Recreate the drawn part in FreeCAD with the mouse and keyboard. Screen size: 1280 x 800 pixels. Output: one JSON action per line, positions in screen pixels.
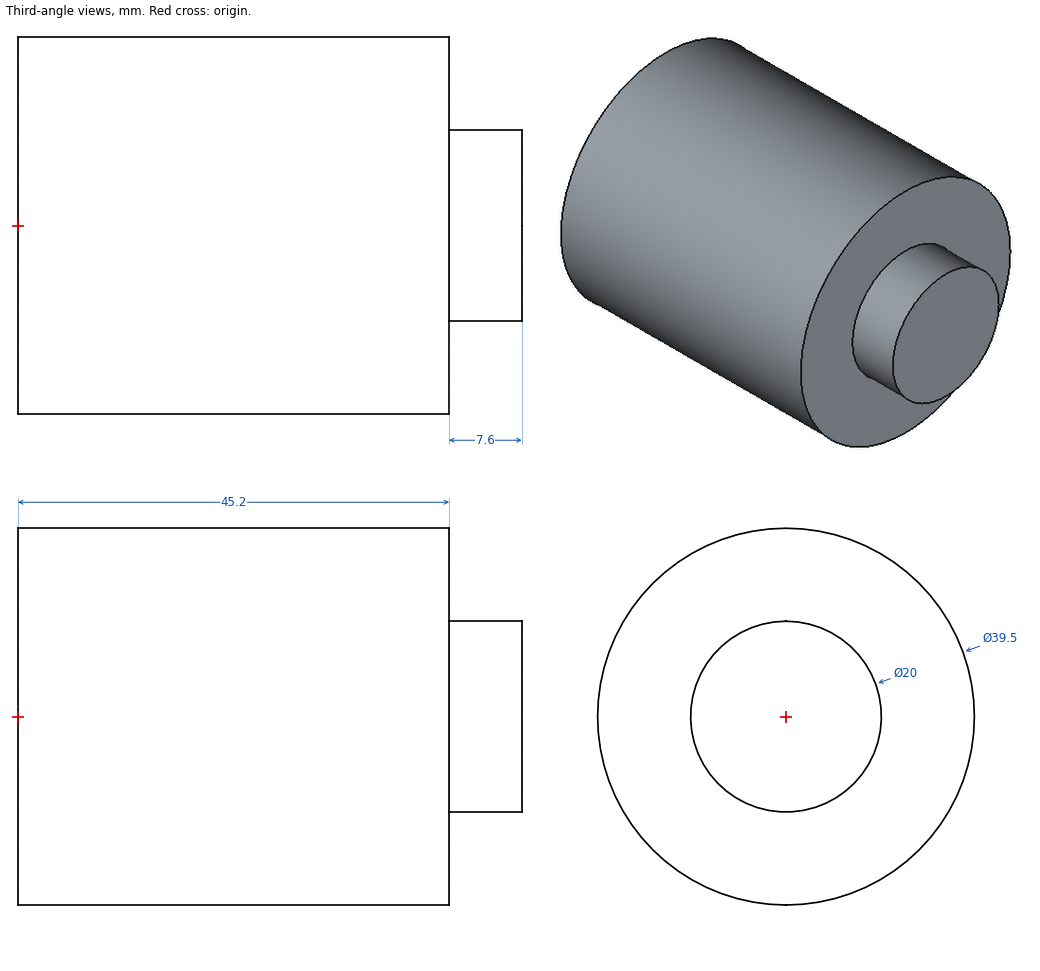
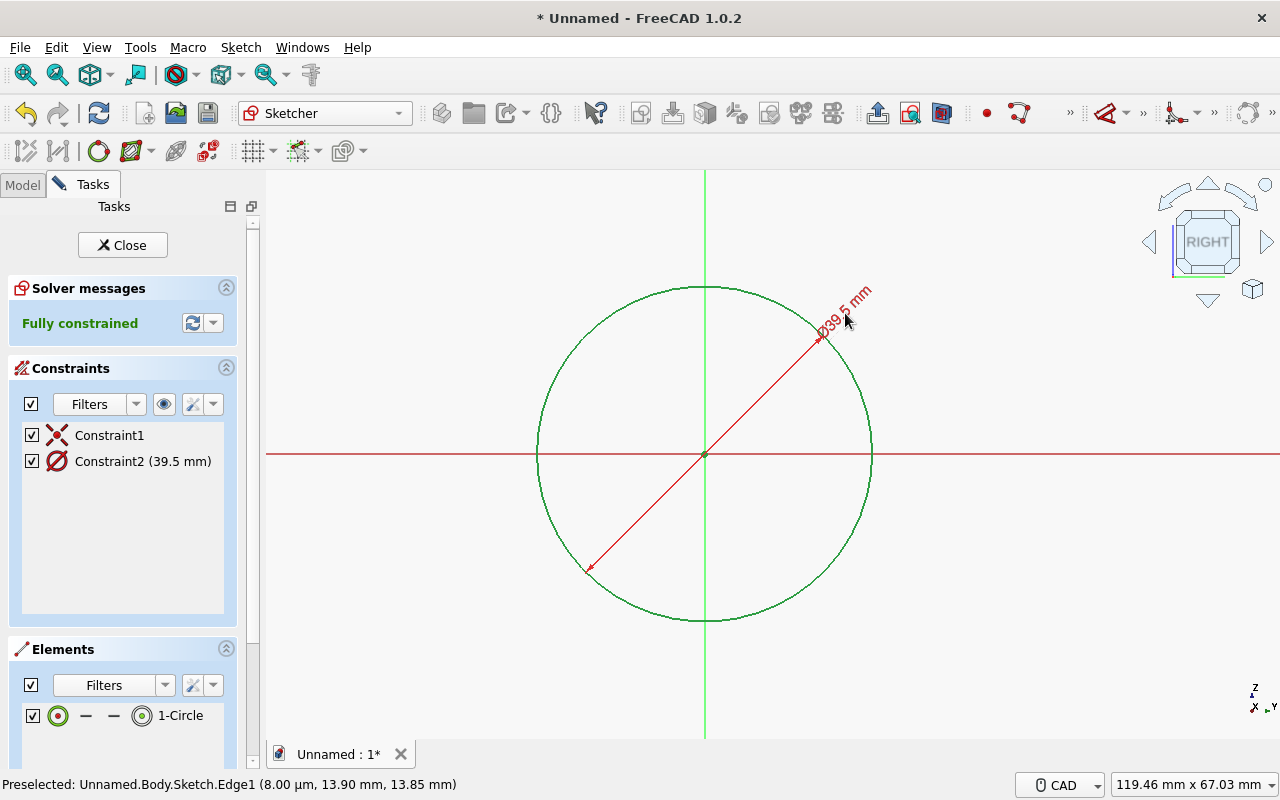
{"action": "left_click", "coordinate": [123, 245]}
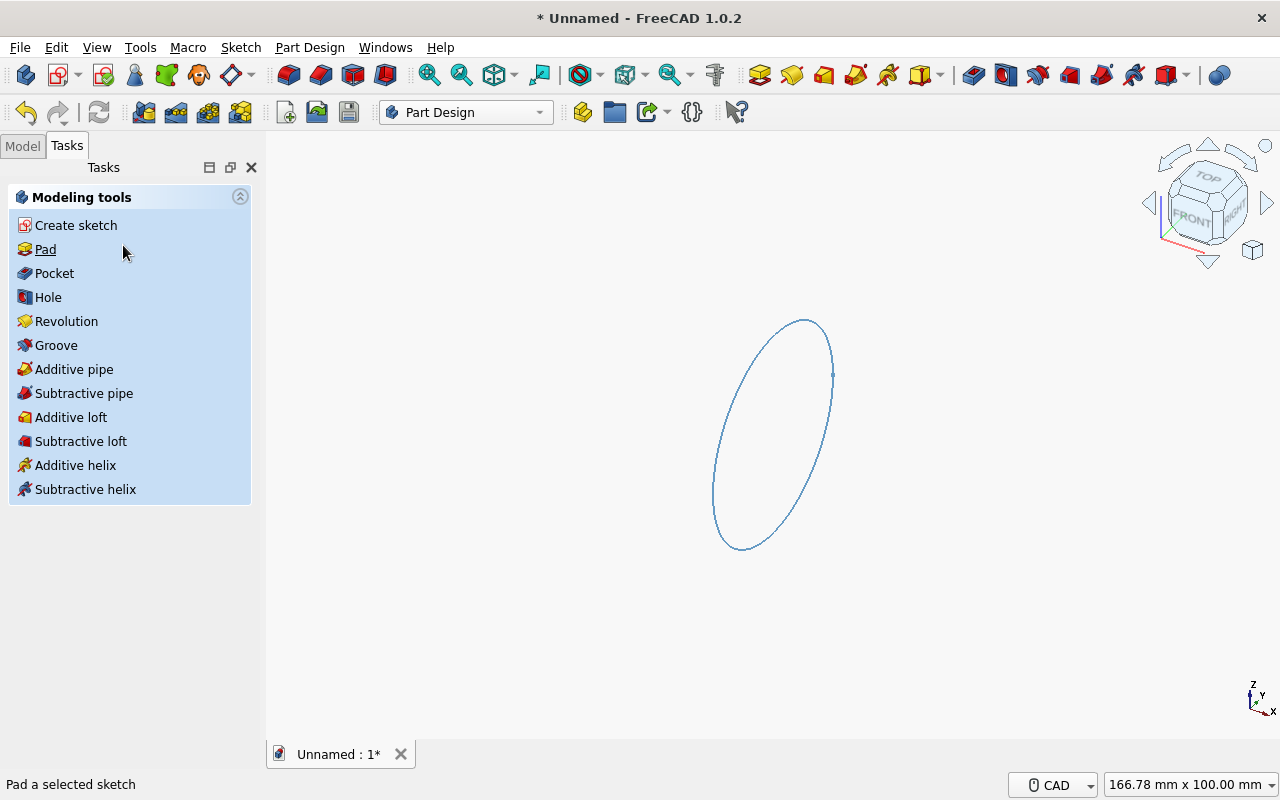
{"action": "left_click", "coordinate": [760, 76]}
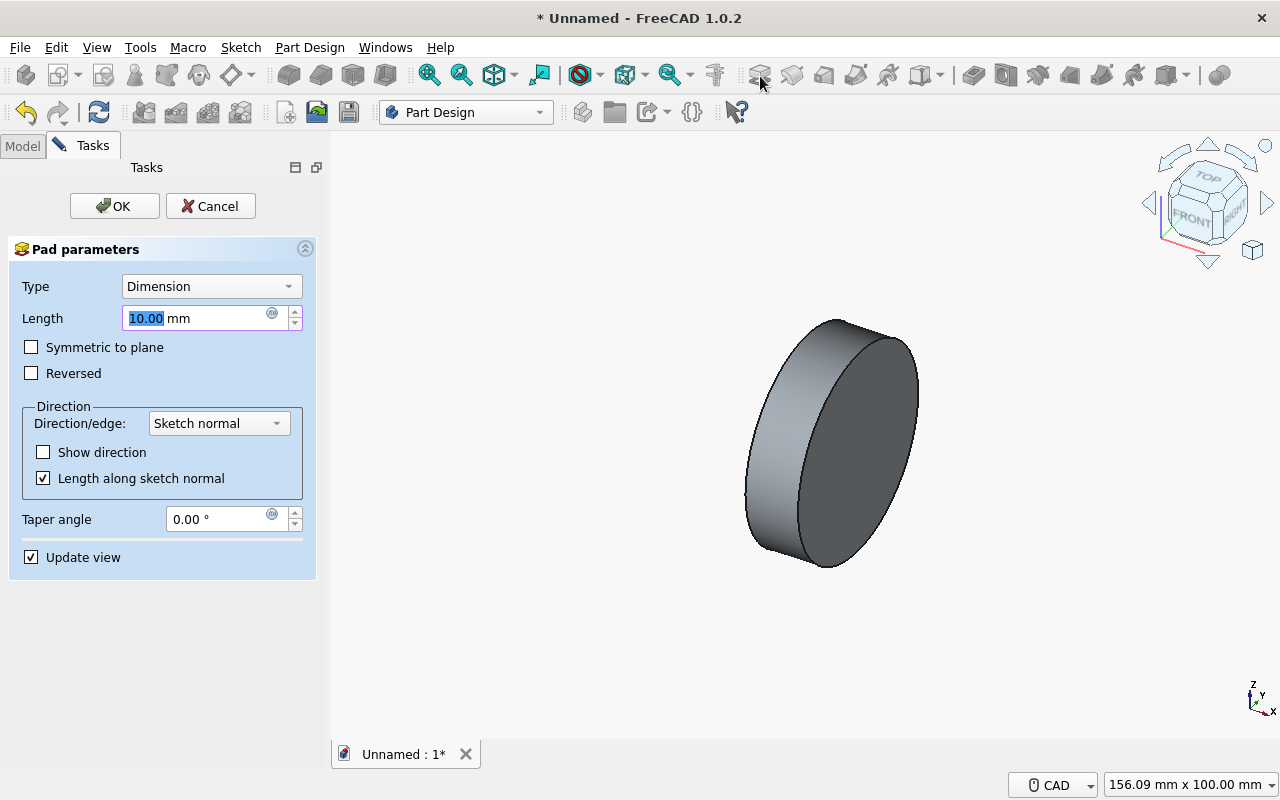
{"action": "type", "text": "45.2"}
{"action": "key", "text": "Tab"}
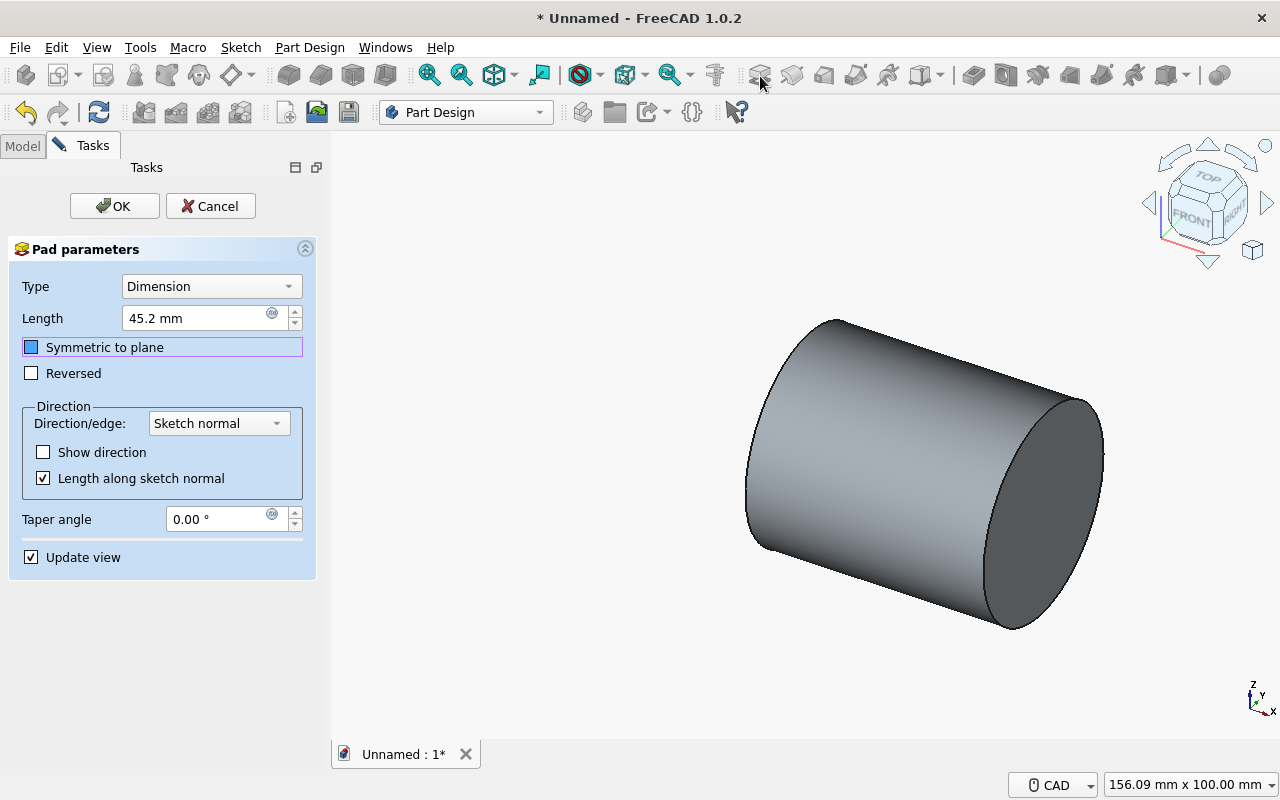
{"action": "left_click", "coordinate": [115, 206]}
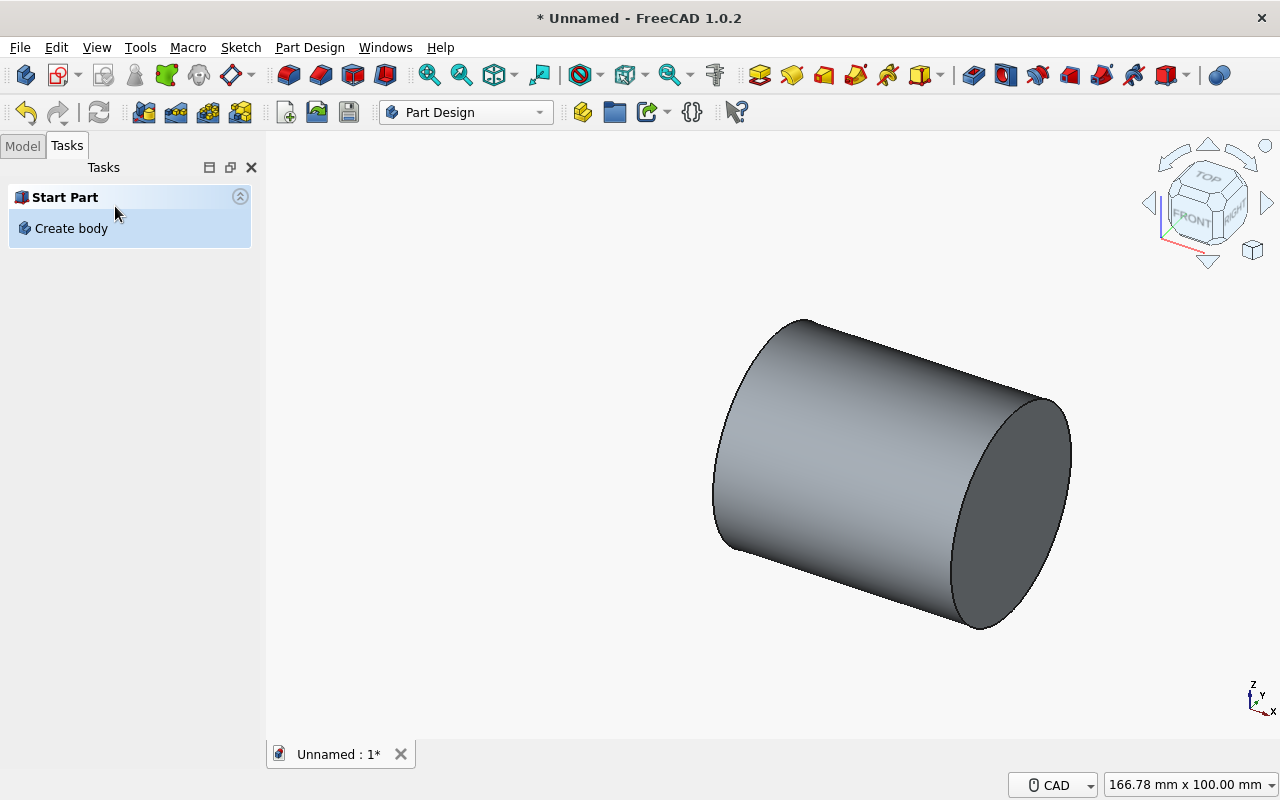
{"action": "left_click", "coordinate": [1011, 513]}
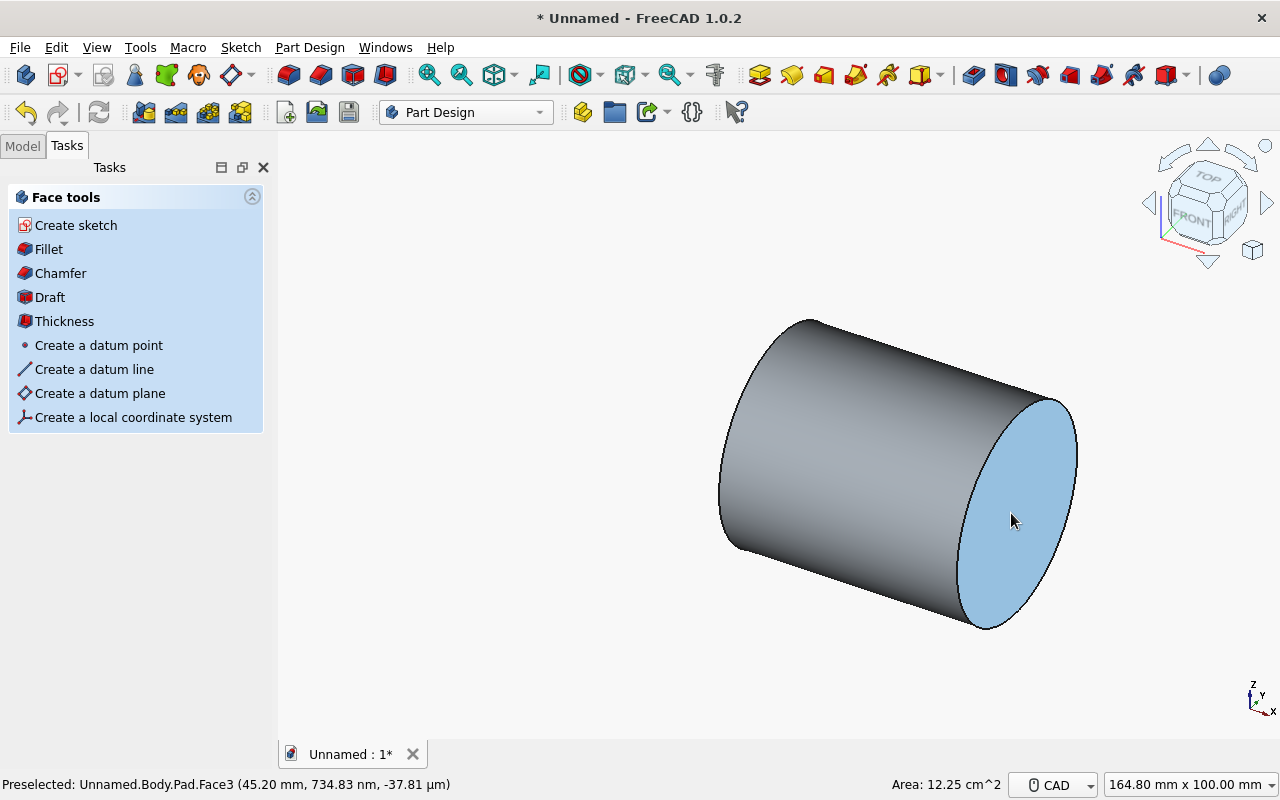
{"action": "left_click", "coordinate": [58, 76]}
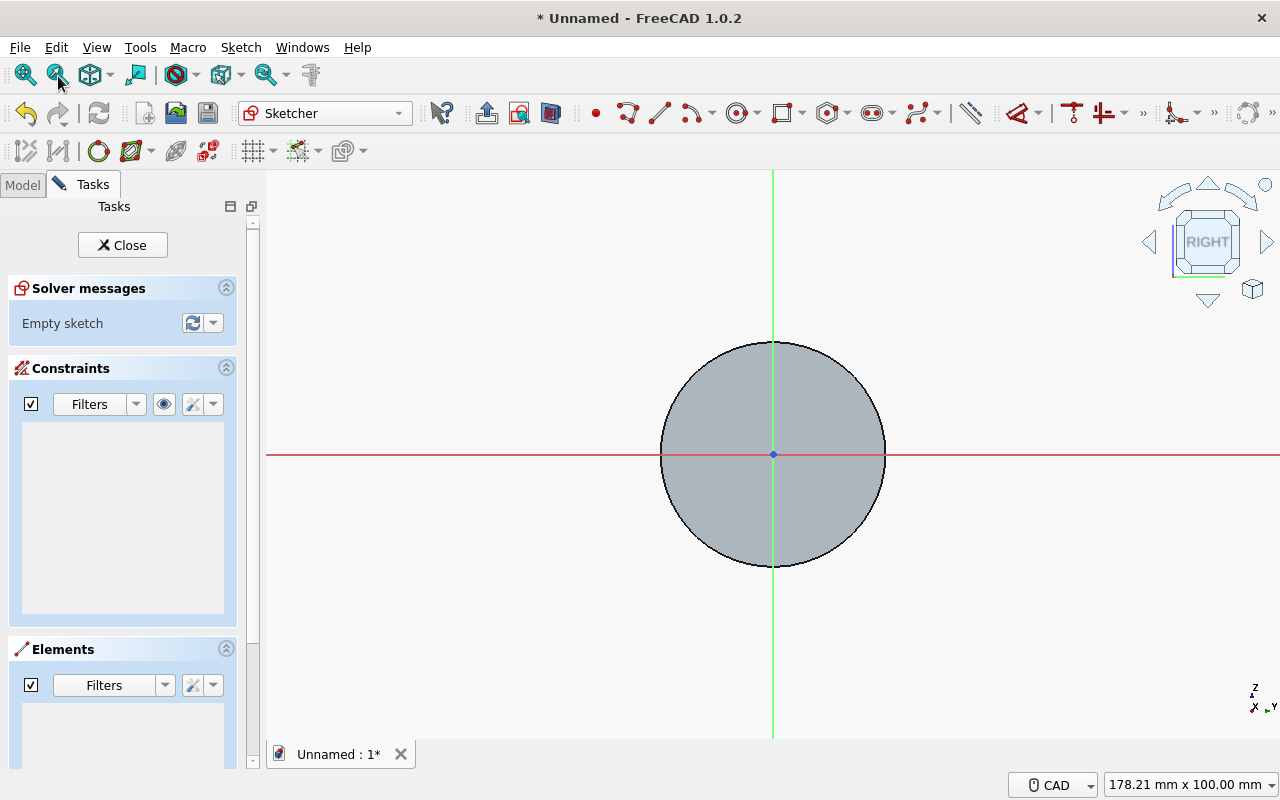
{"action": "scroll", "coordinate": [803, 454], "scroll_direction": "up", "scroll_amount": 6}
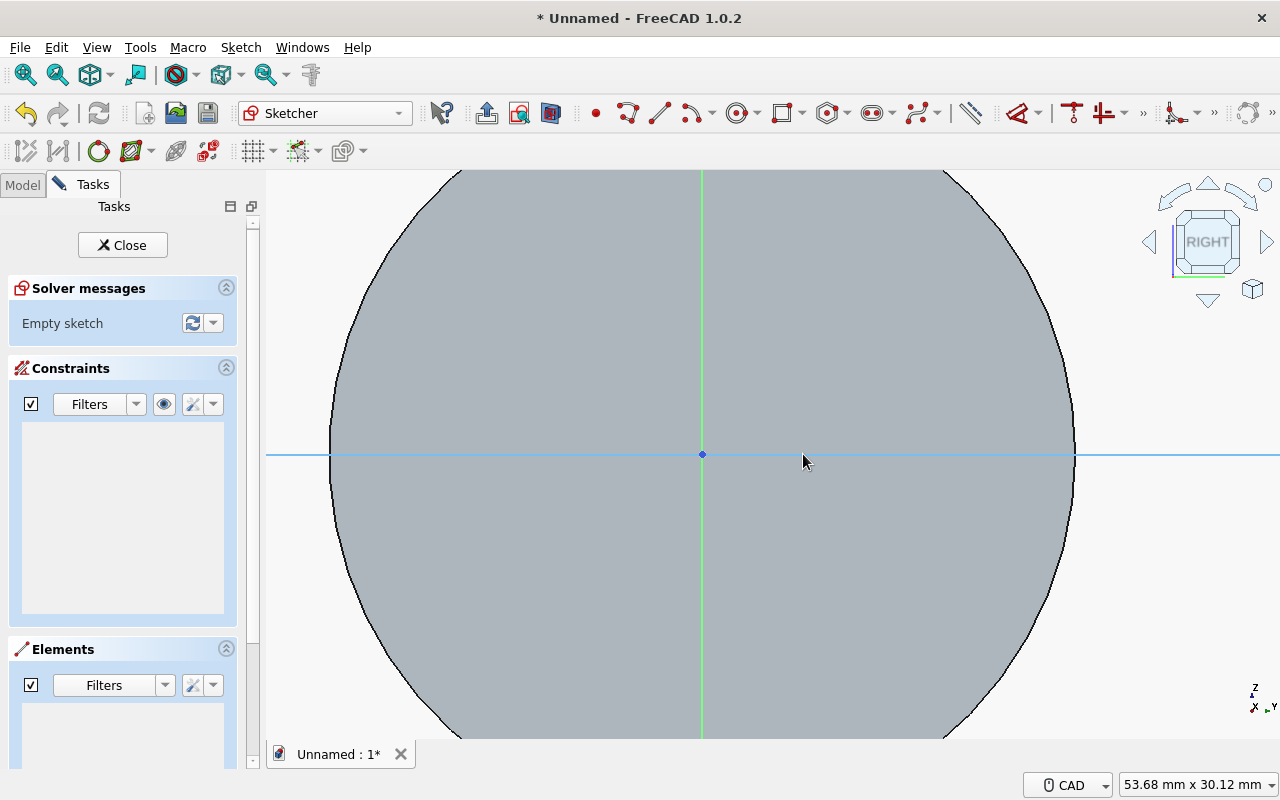
{"action": "left_click", "coordinate": [738, 114]}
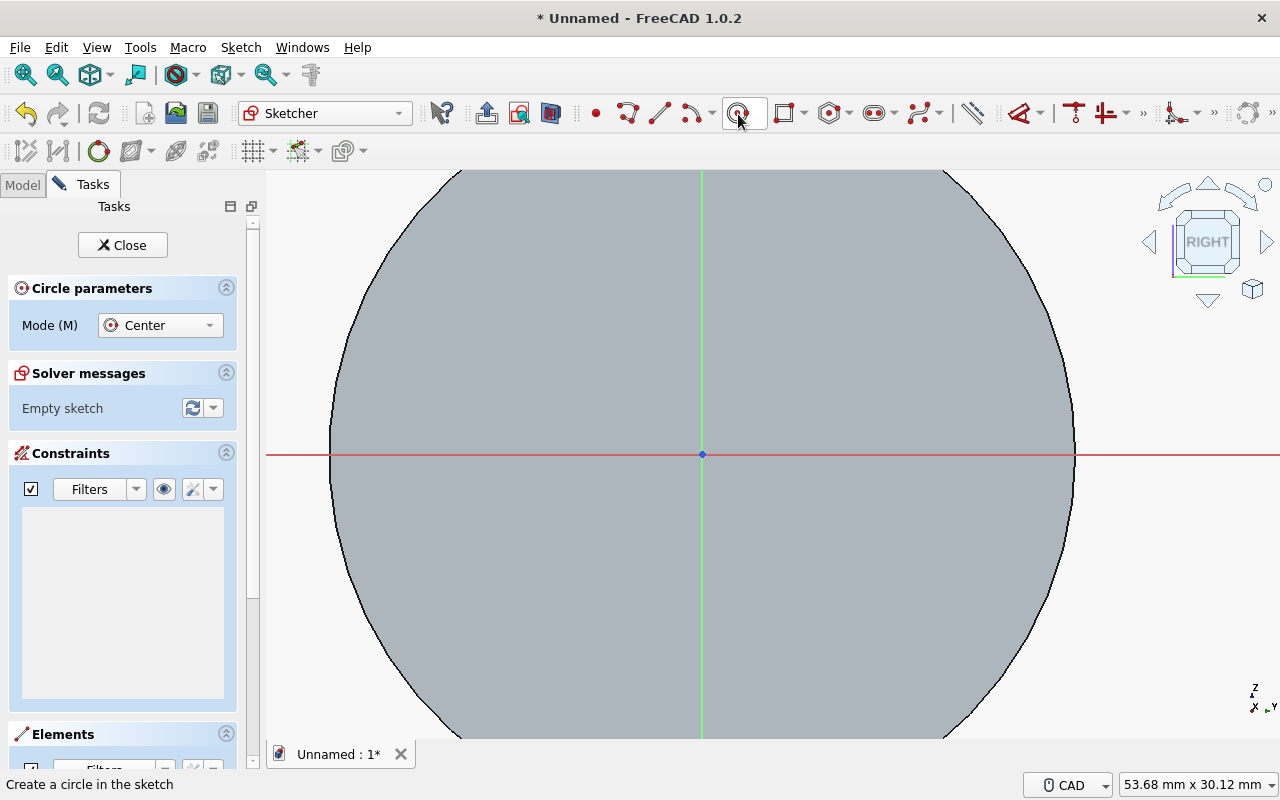
{"action": "left_click", "coordinate": [702, 454]}
{"action": "left_click", "coordinate": [836, 321]}
{"action": "key", "text": "Escape"}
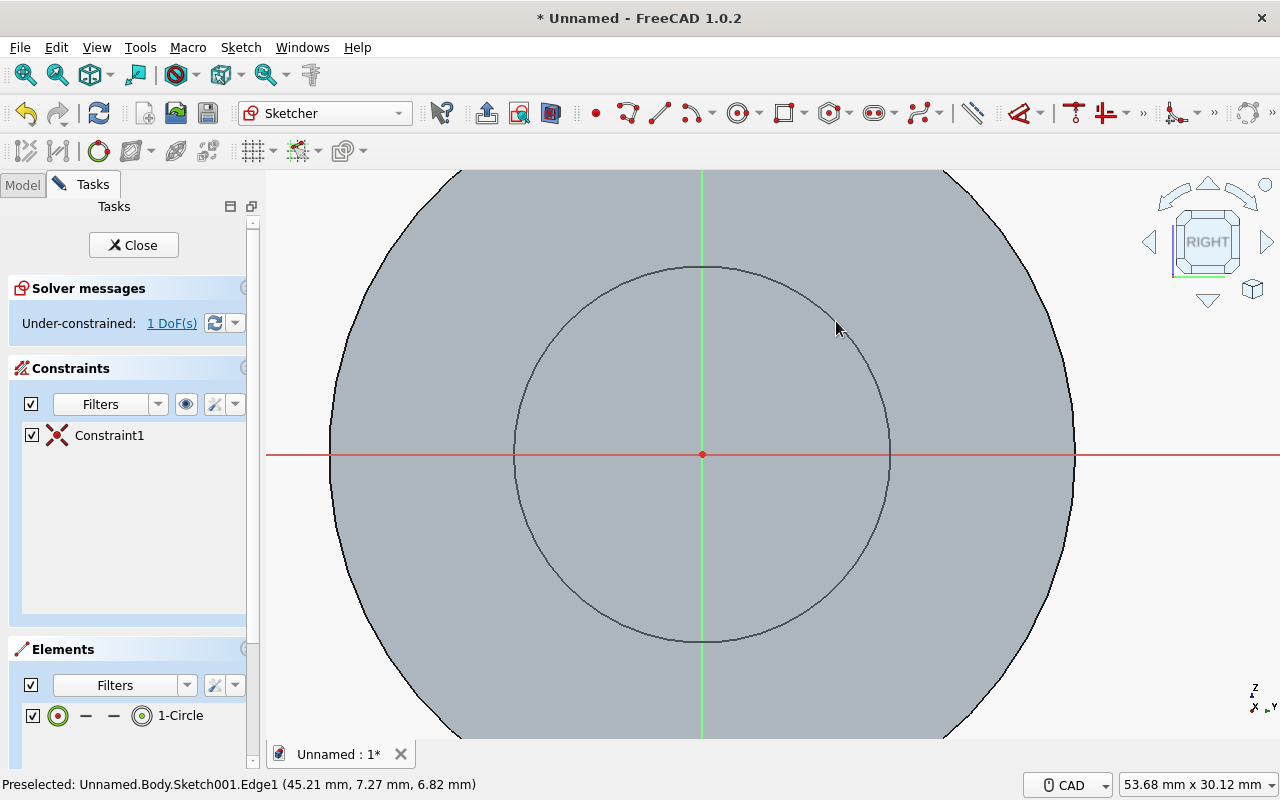
{"action": "left_click", "coordinate": [1020, 114]}